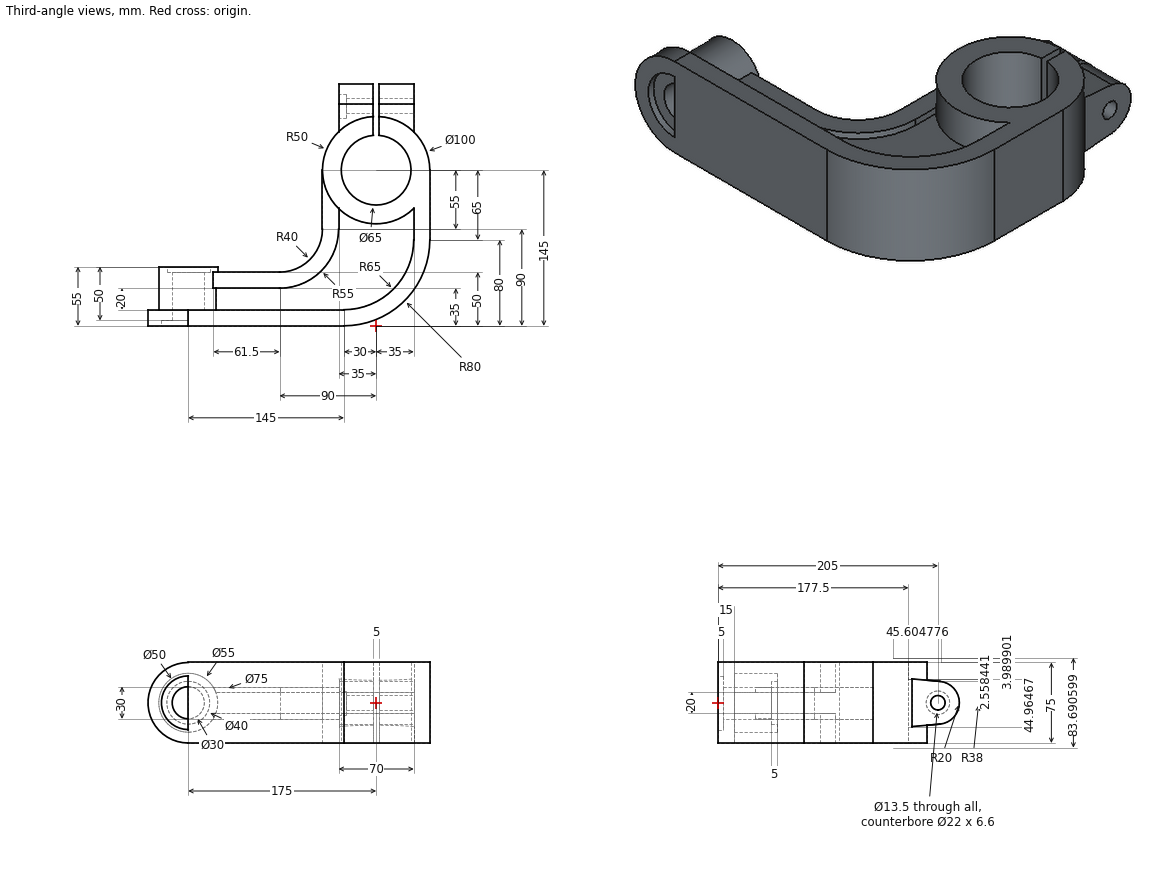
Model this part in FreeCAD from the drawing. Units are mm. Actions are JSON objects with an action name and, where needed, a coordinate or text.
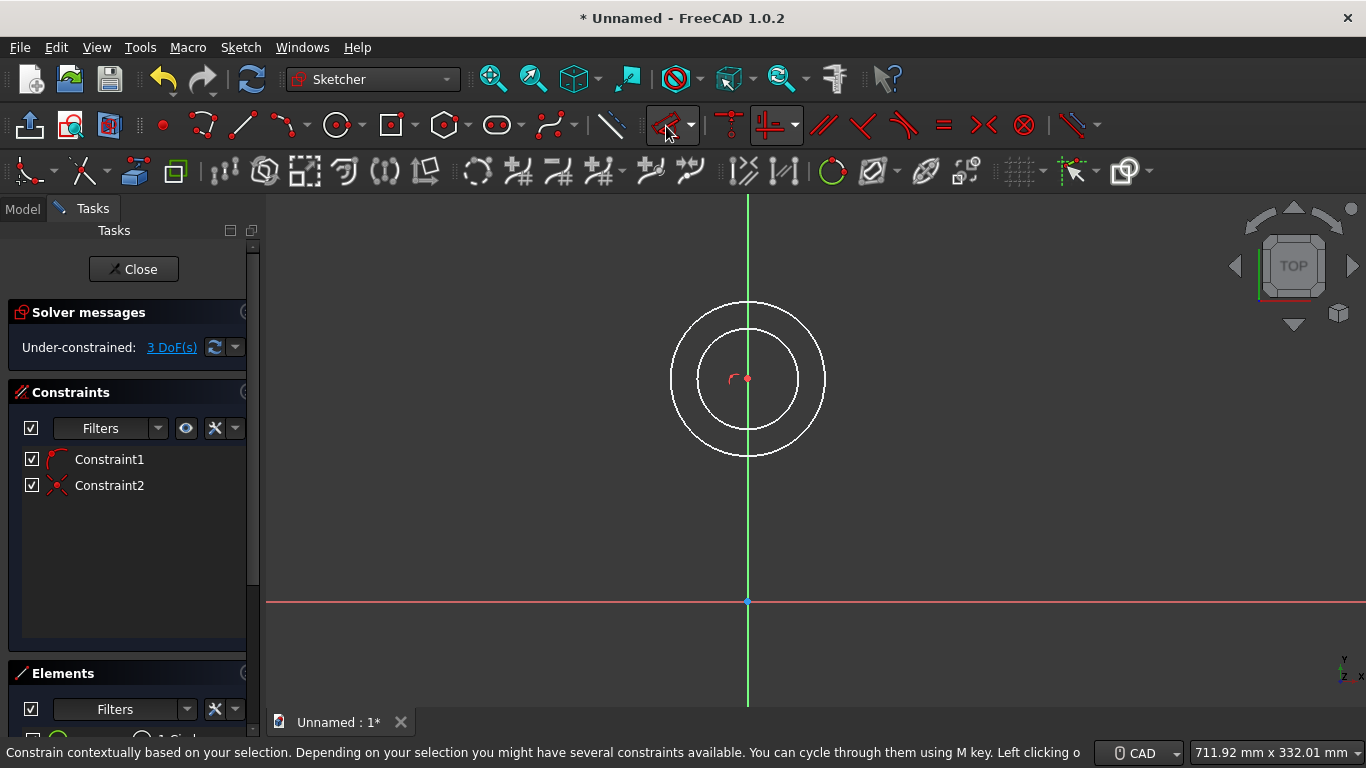
{"action": "left_click", "coordinate": [802, 324]}
{"action": "left_click", "coordinate": [824, 301]}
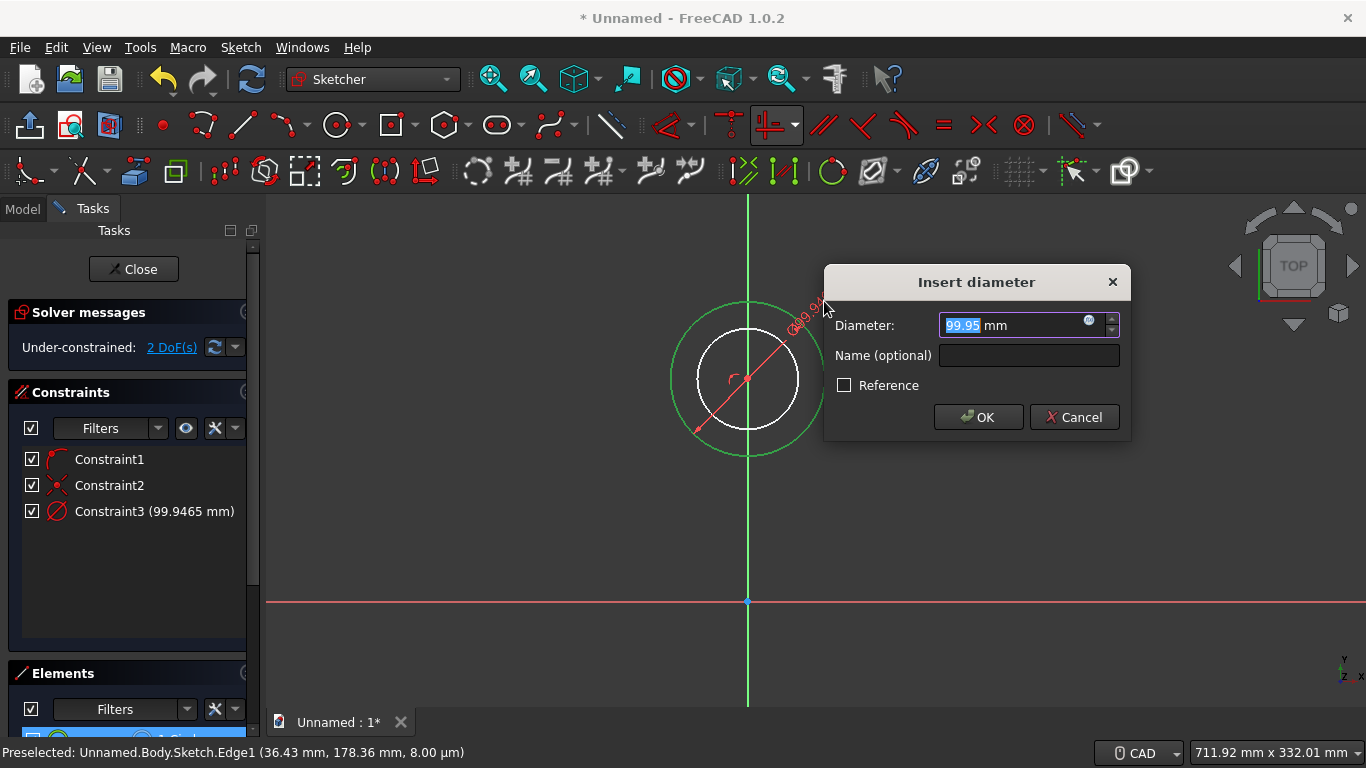
{"action": "type", "text": "100"}
{"action": "key", "text": "Return"}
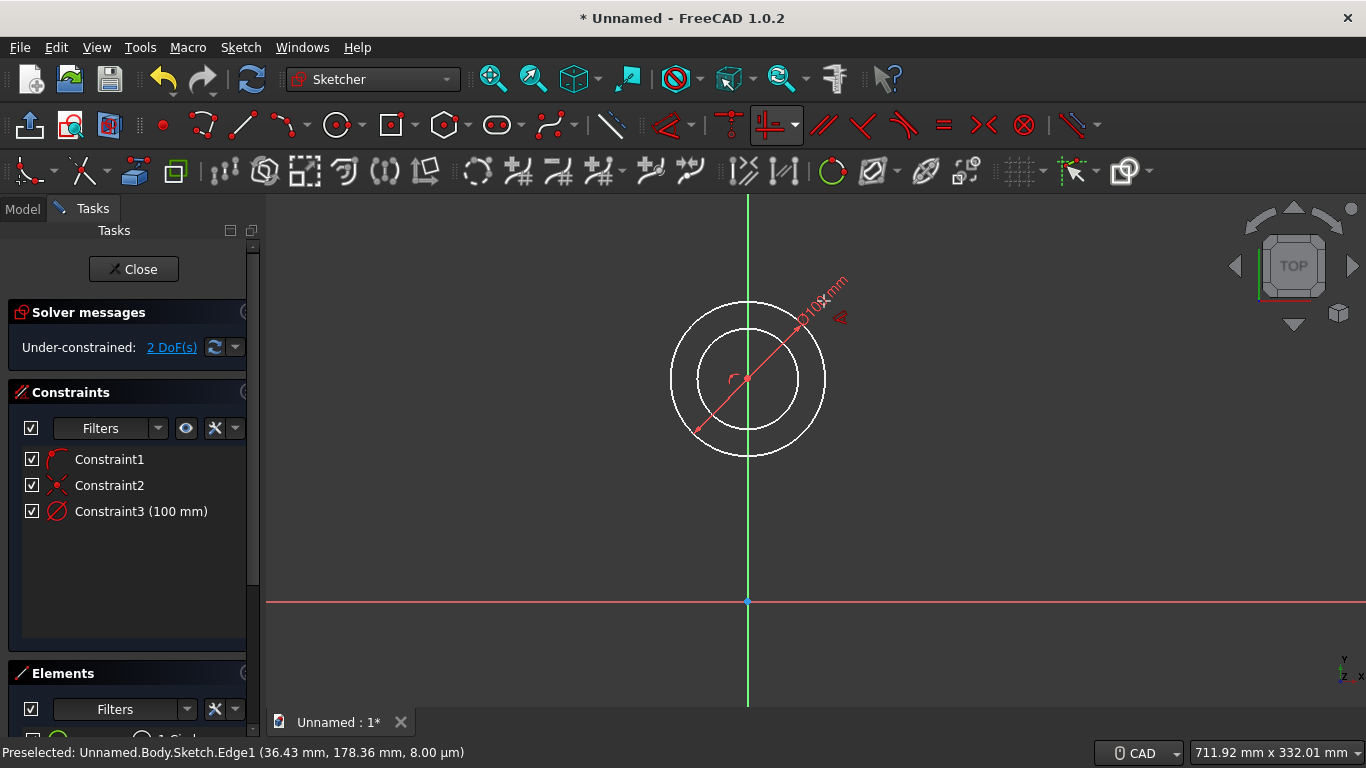
{"action": "left_click", "coordinate": [783, 343]}
{"action": "left_click", "coordinate": [849, 348]}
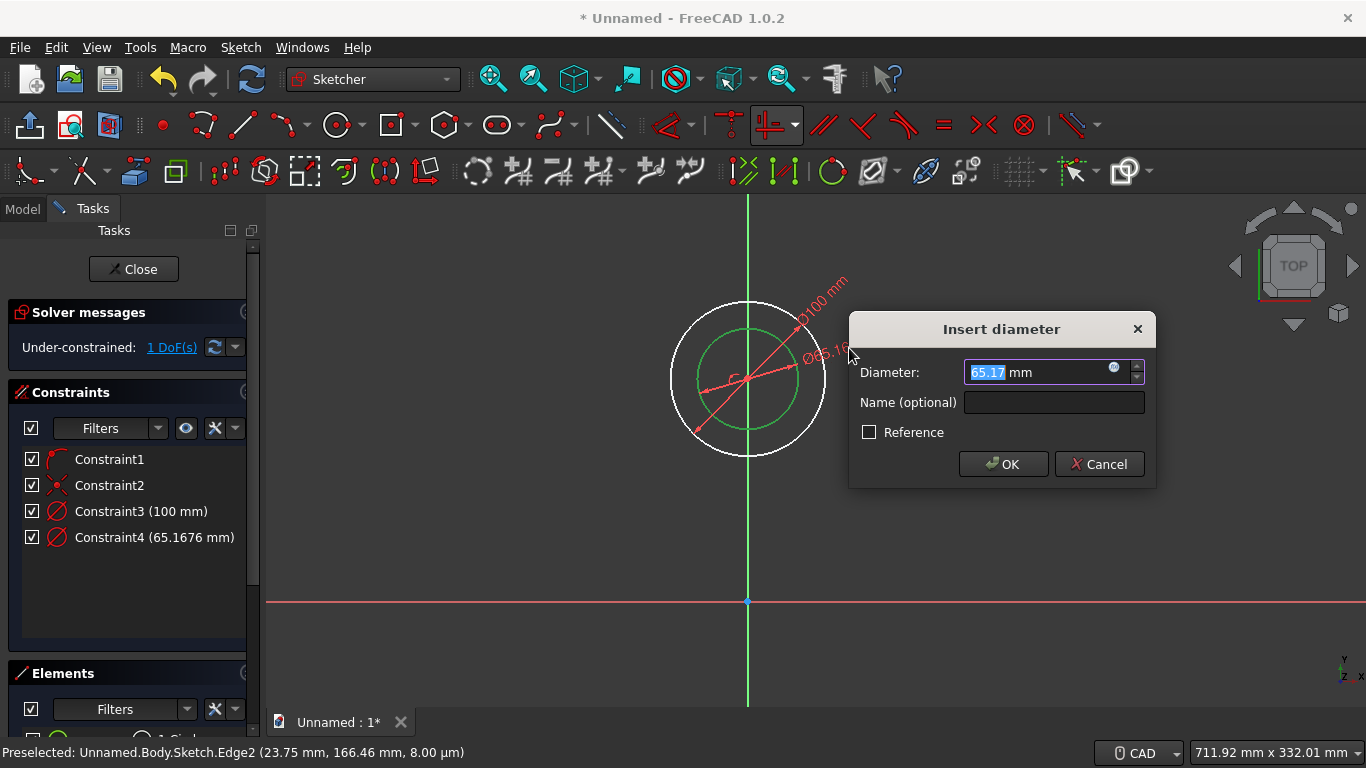
{"action": "type", "text": "65"}
{"action": "key", "text": "Return"}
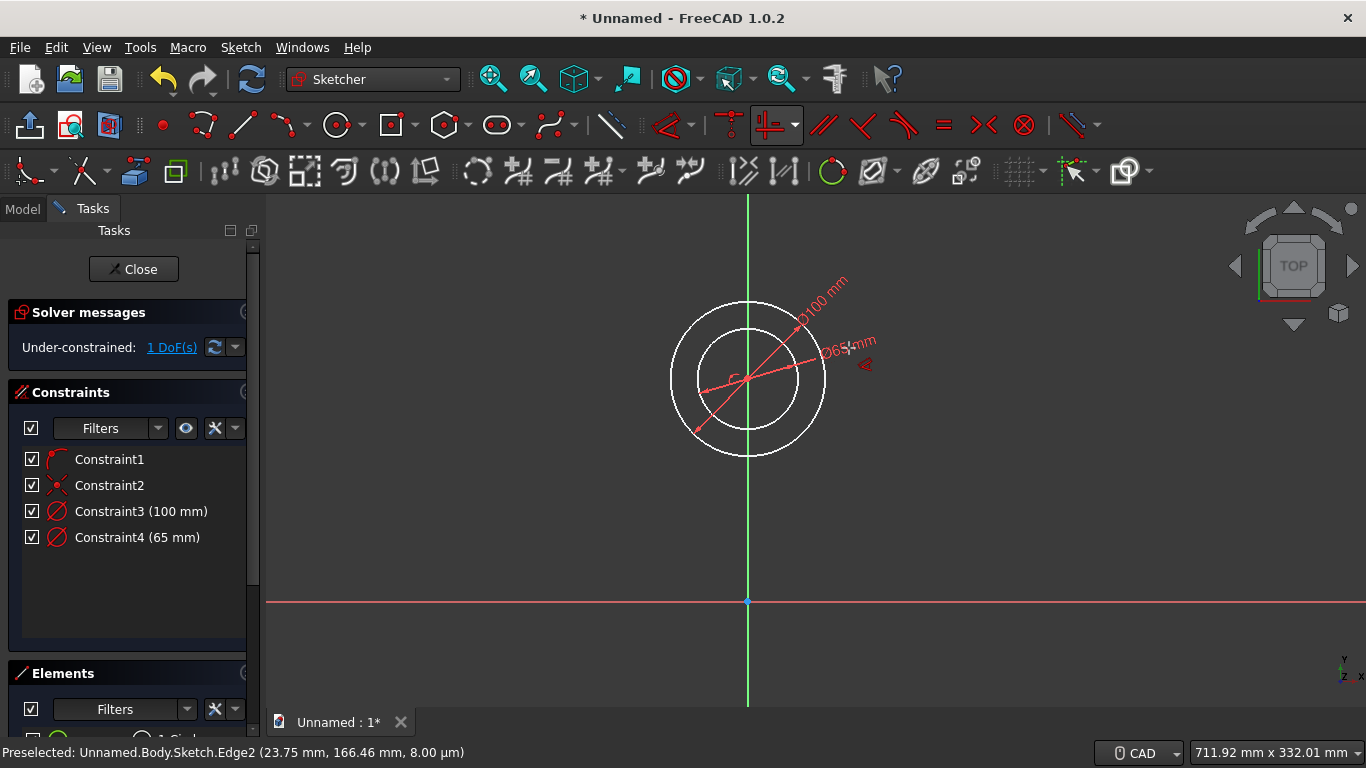
{"action": "left_click", "coordinate": [748, 379]}
{"action": "left_click", "coordinate": [782, 490]}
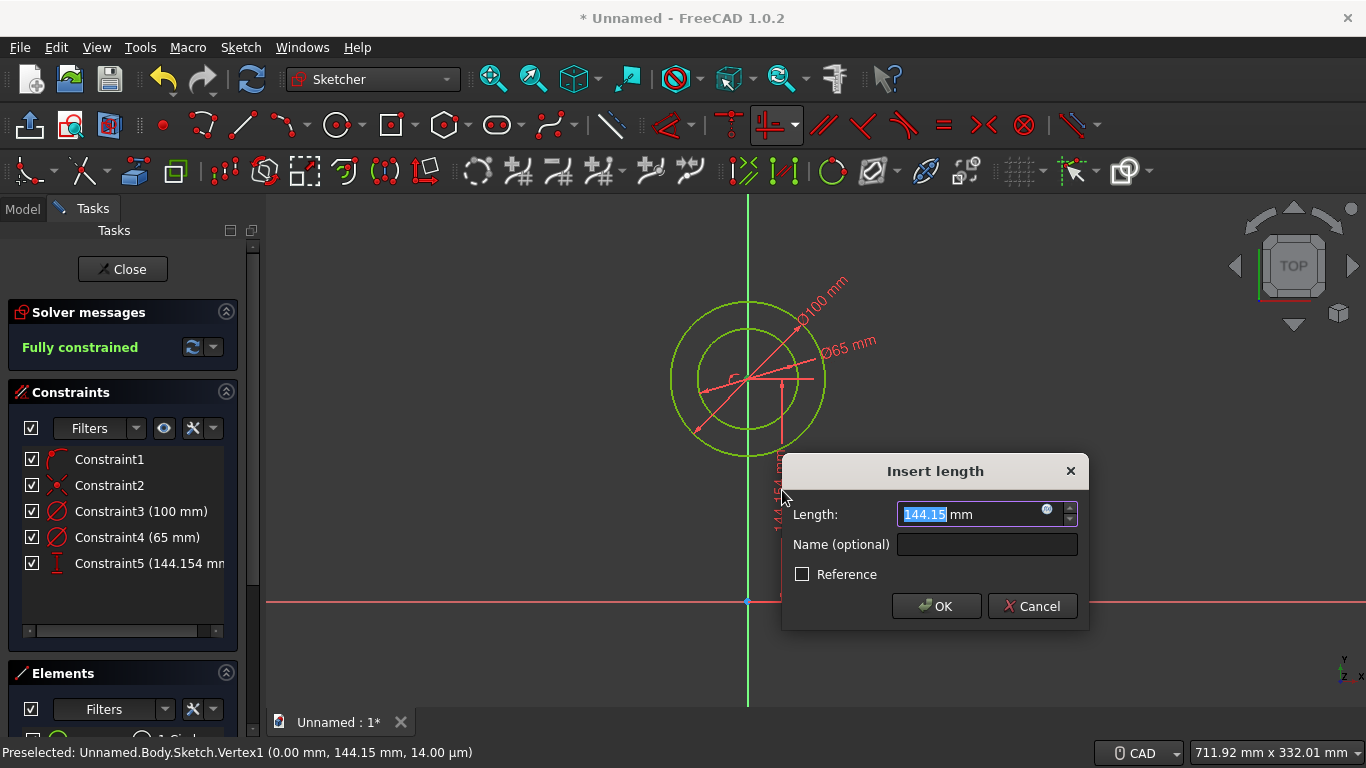
{"action": "type", "text": "145"}
{"action": "key", "text": "Return"}
{"action": "key", "text": "Escape"}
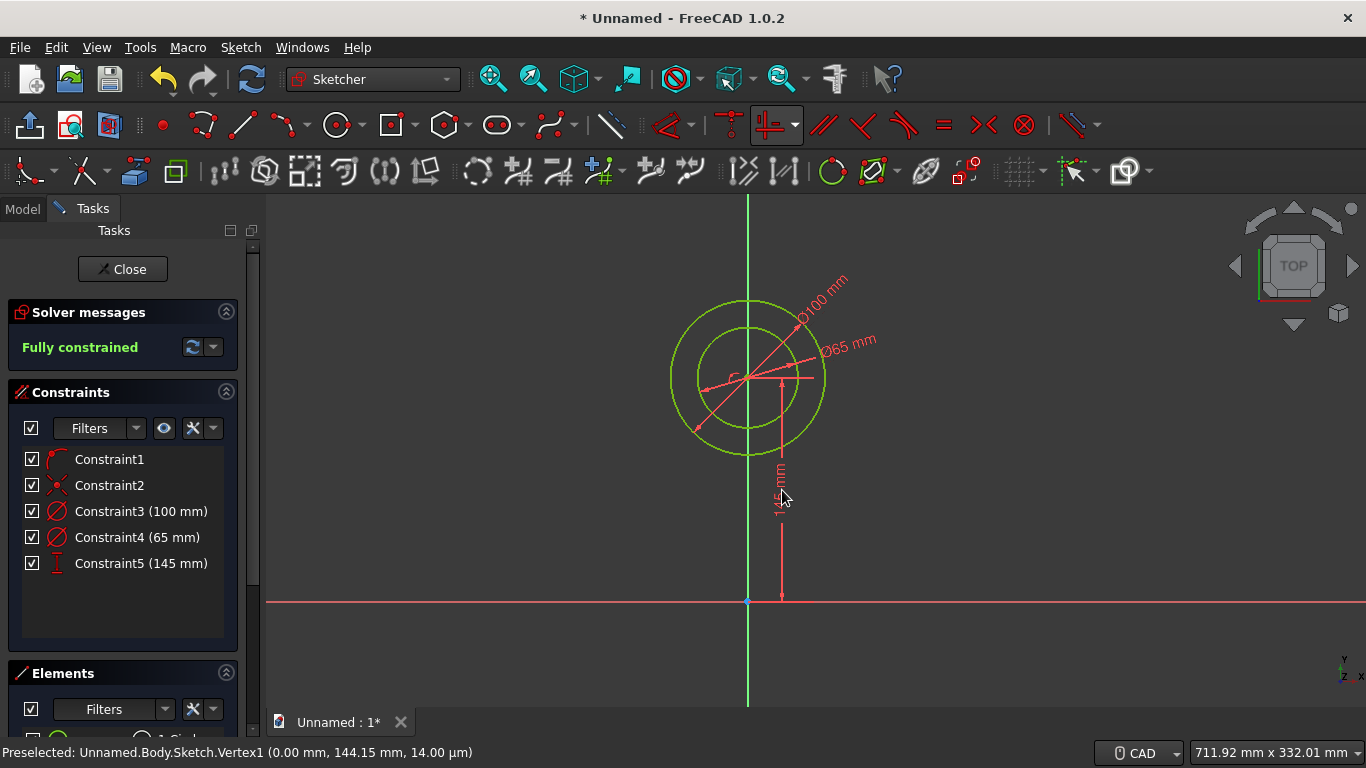
{"action": "left_click", "coordinate": [123, 269]}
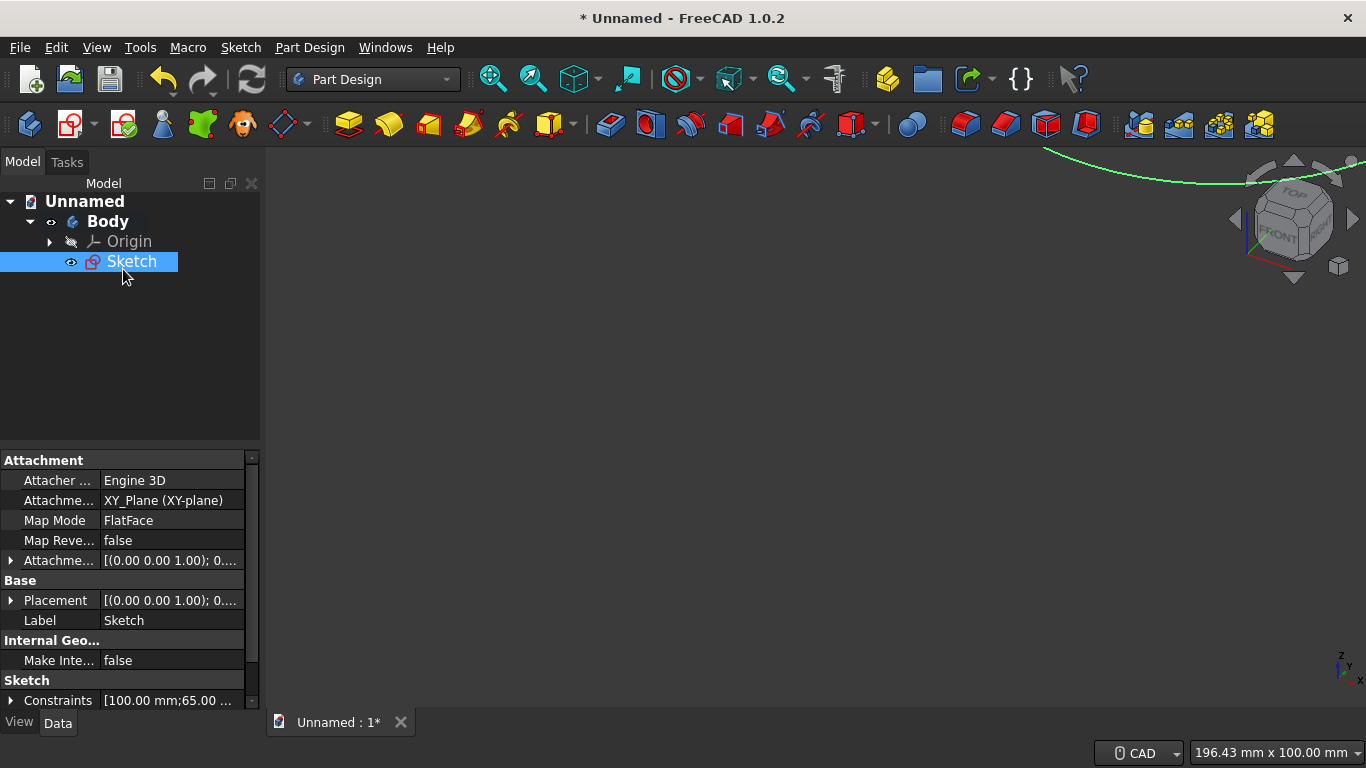
{"action": "left_click", "coordinate": [350, 124]}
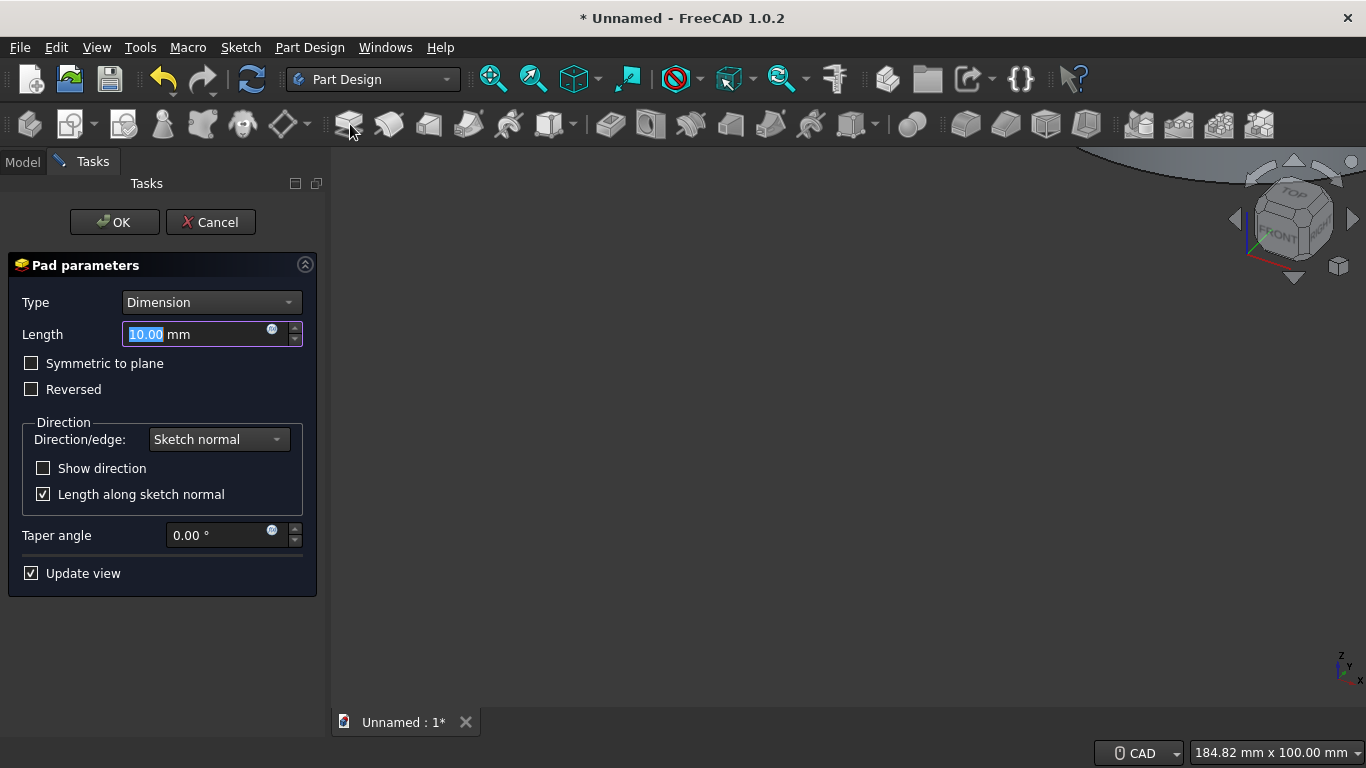
{"action": "type", "text": "75"}
{"action": "key", "text": "Tab"}